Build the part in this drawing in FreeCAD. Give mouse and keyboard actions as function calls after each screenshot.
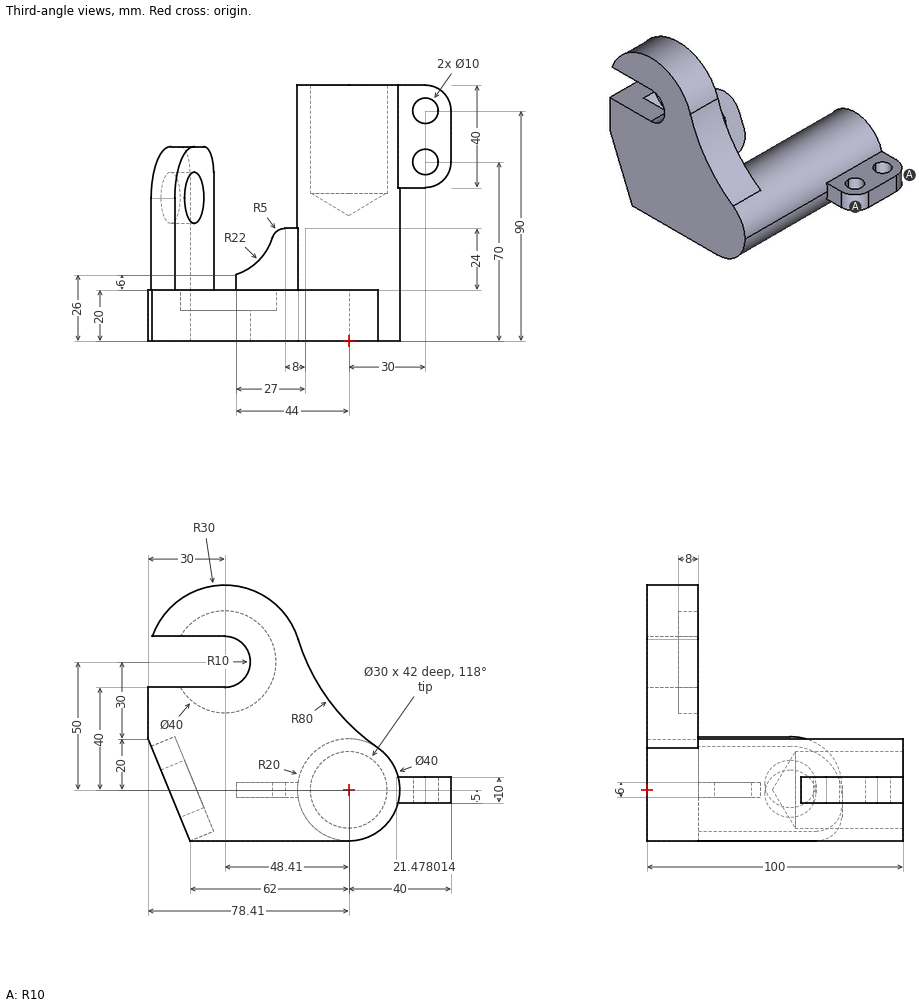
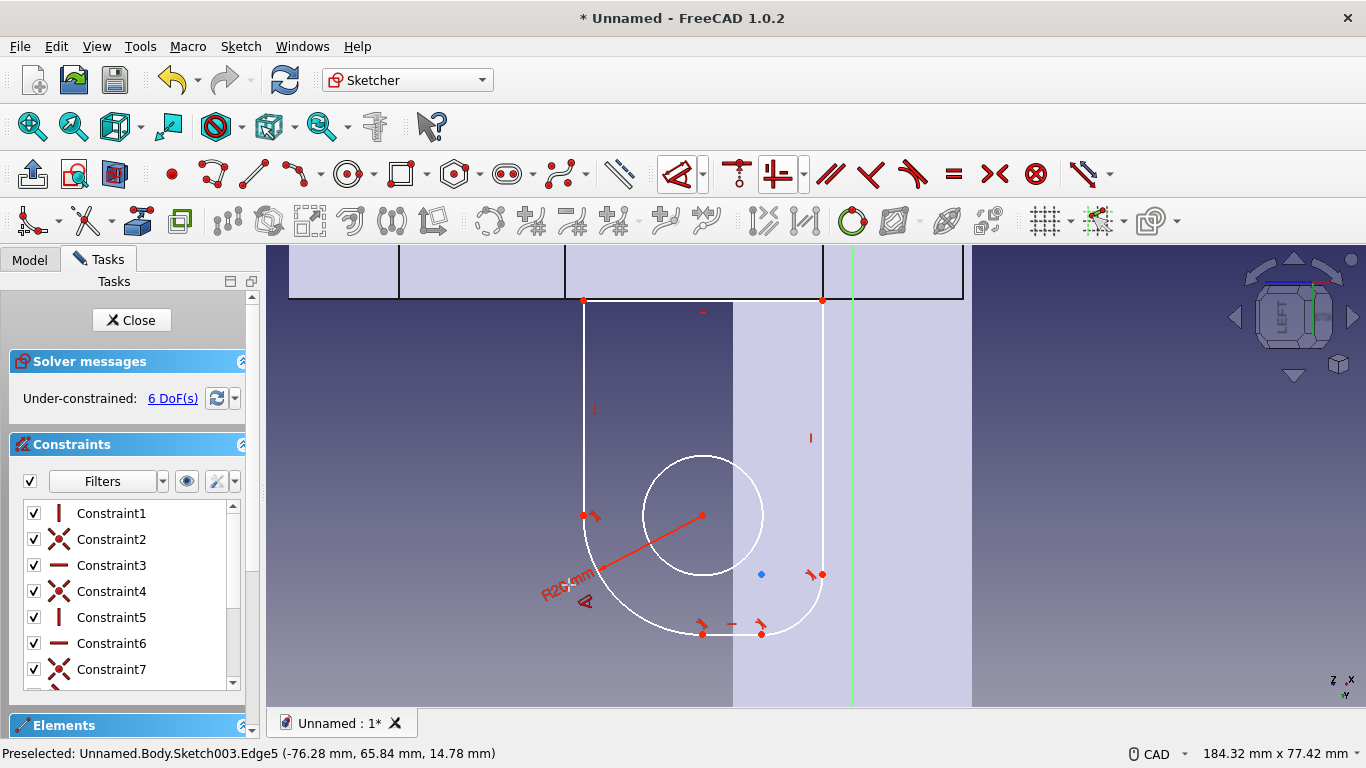
click(789, 628)
click(803, 657)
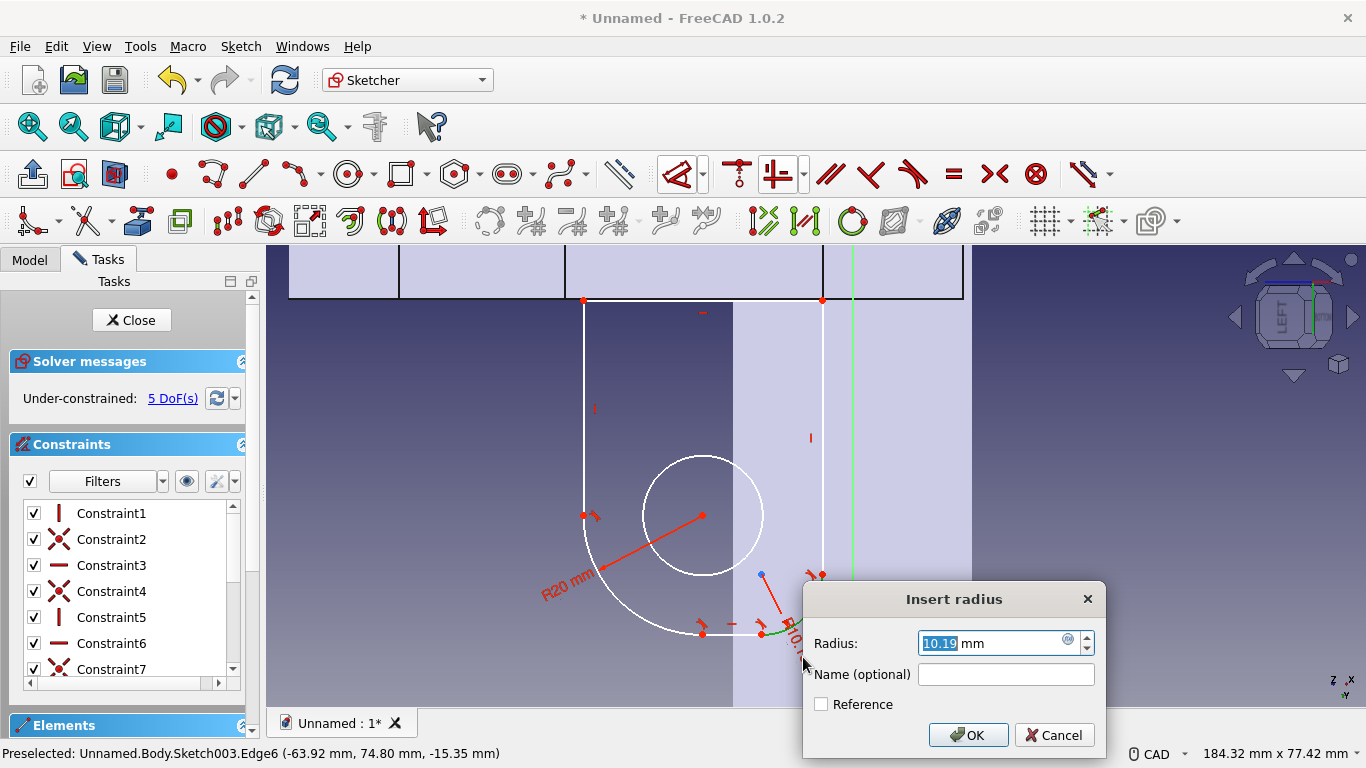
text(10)
key(Return)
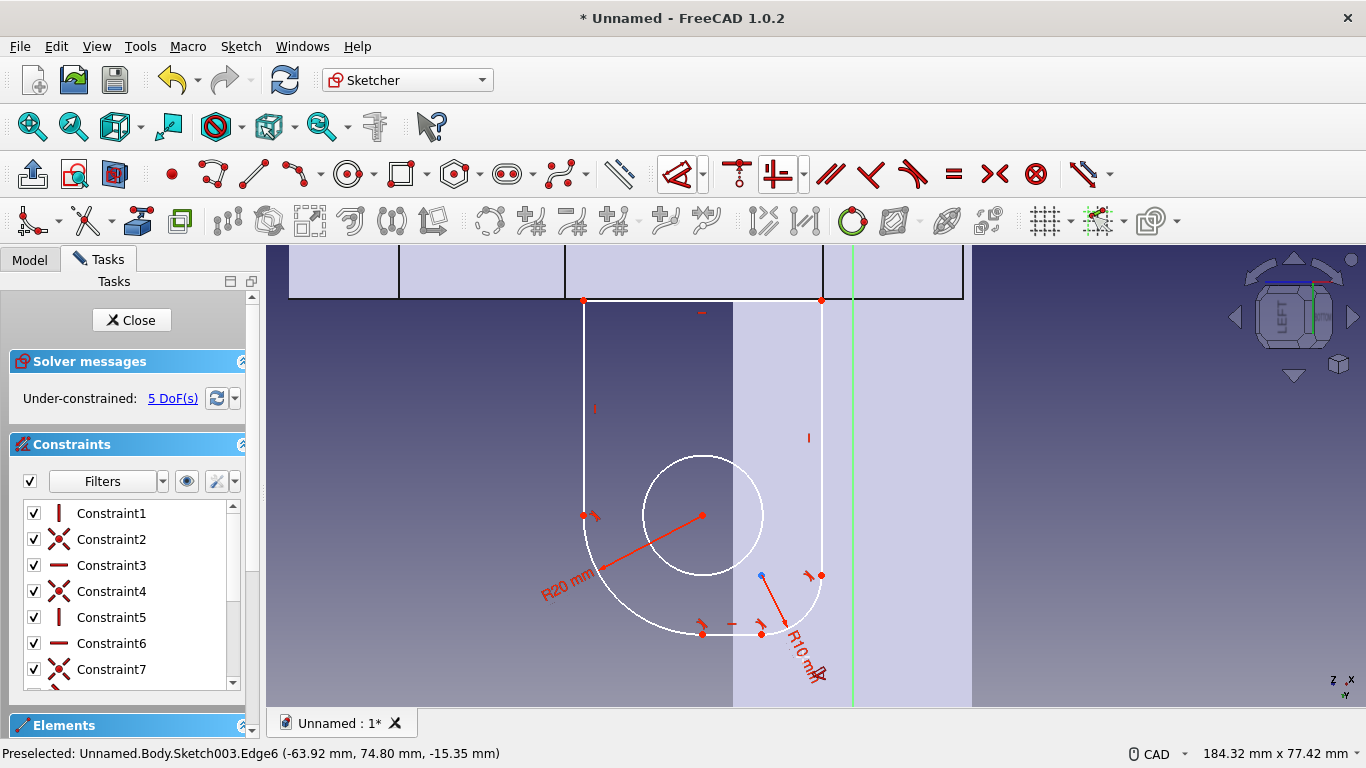
click(745, 473)
click(768, 450)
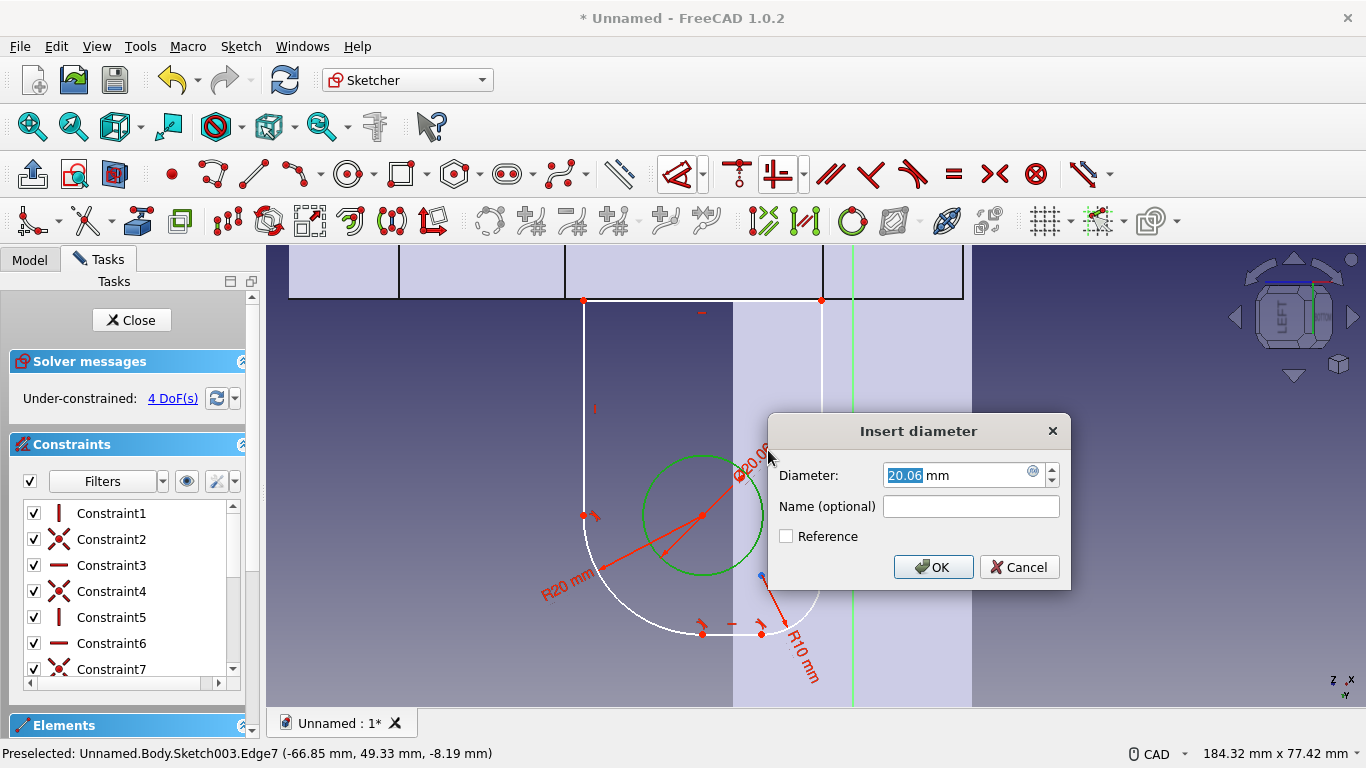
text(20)
key(Return)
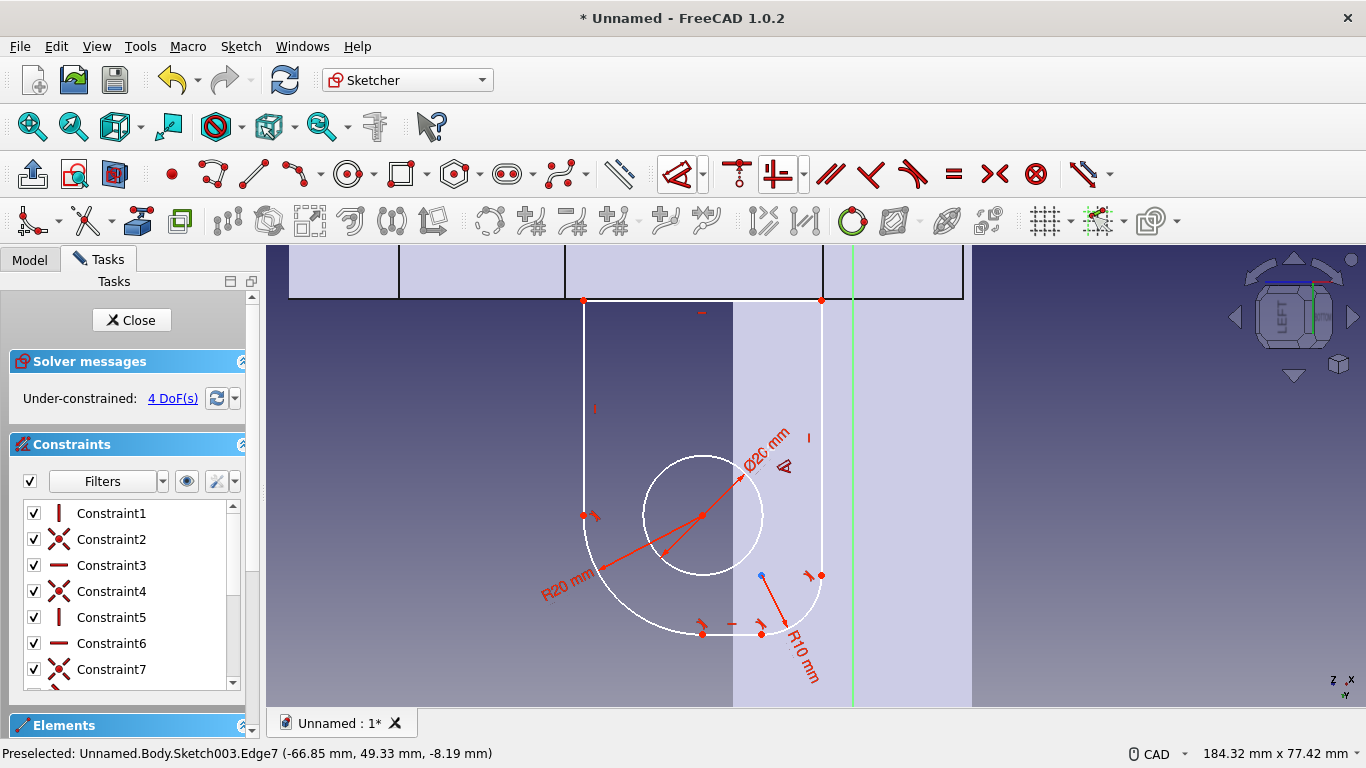
click(822, 493)
click(788, 375)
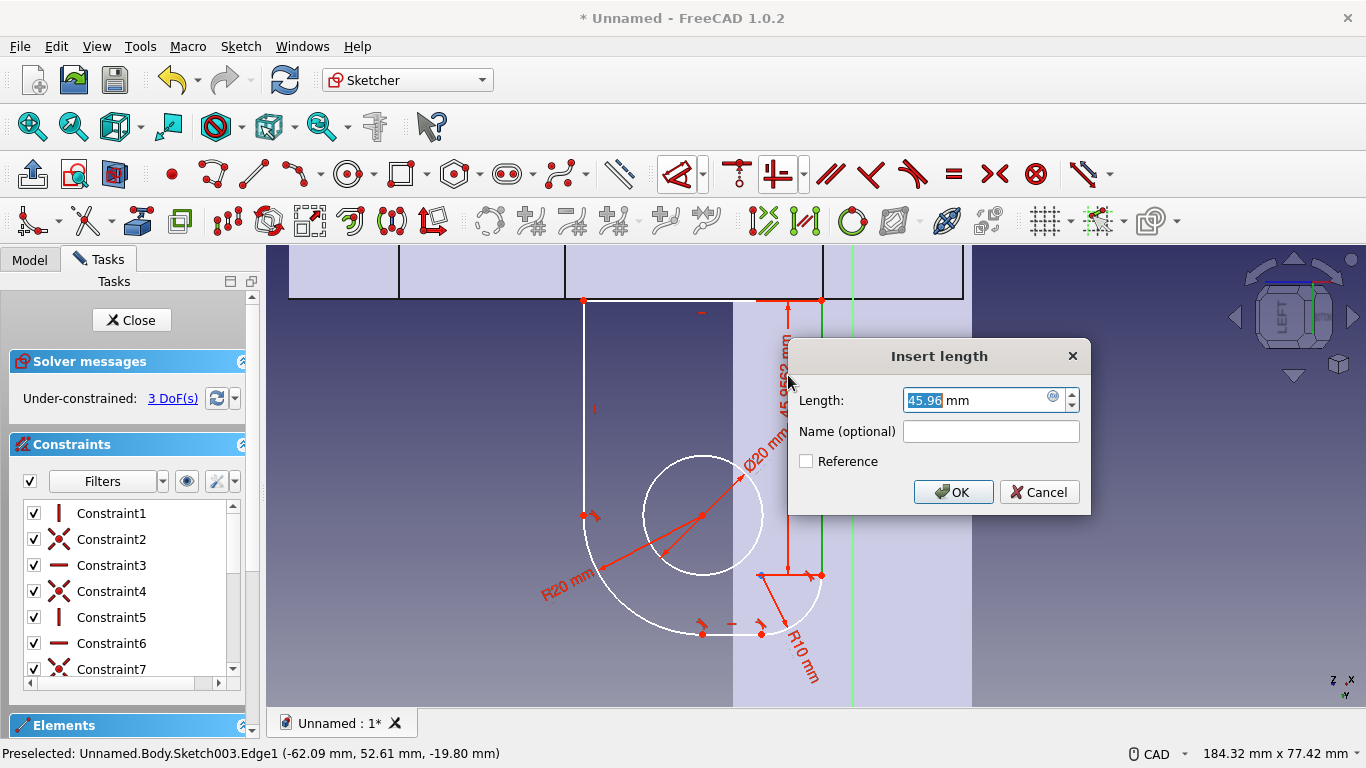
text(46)
key(Return)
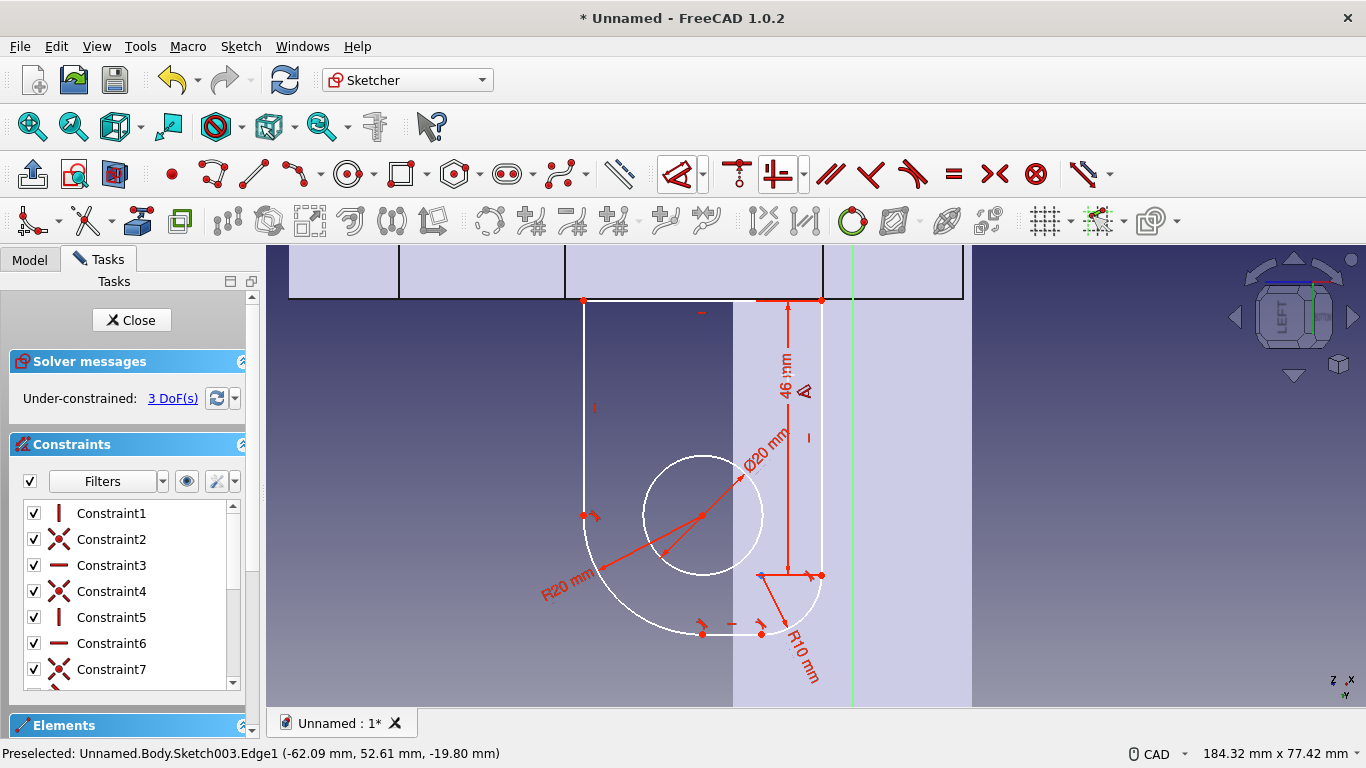
click(750, 301)
click(703, 335)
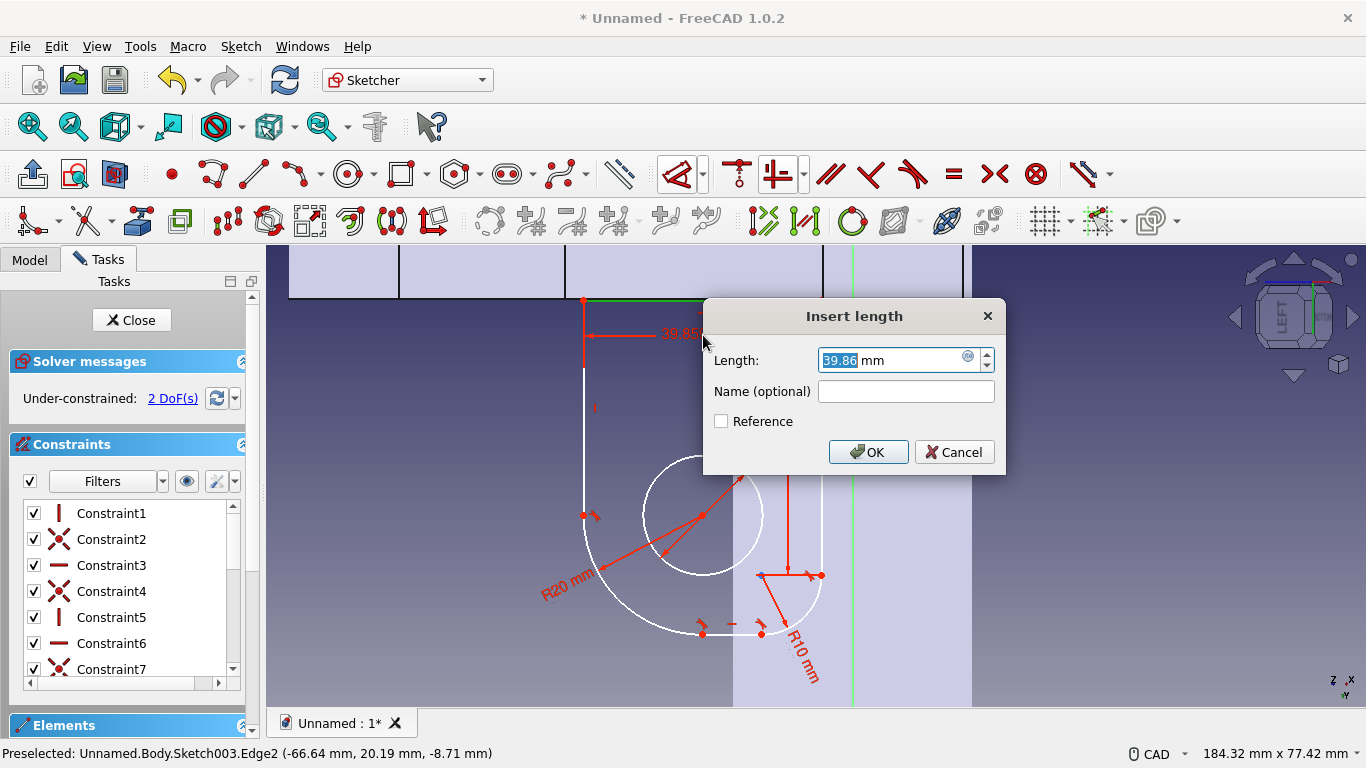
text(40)
key(Return)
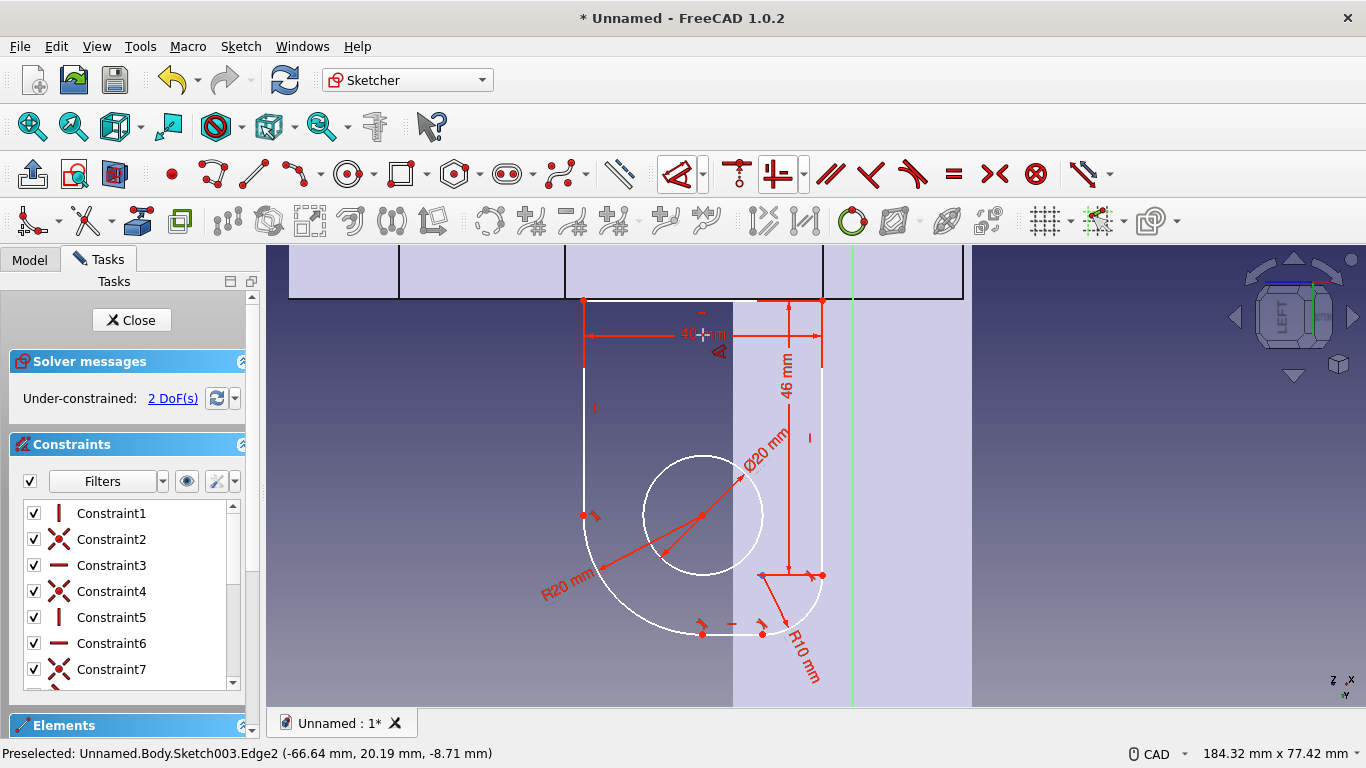
click(703, 515)
click(887, 394)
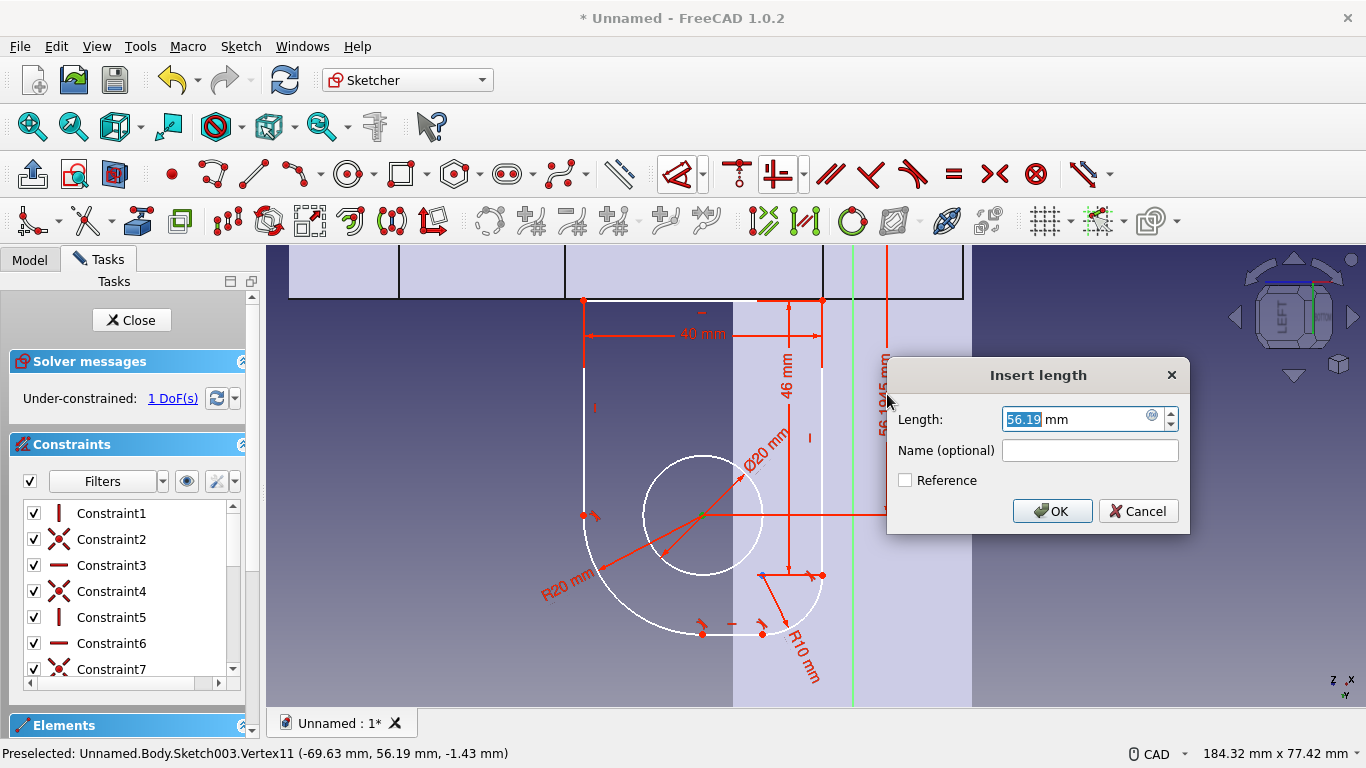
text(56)
key(Return)